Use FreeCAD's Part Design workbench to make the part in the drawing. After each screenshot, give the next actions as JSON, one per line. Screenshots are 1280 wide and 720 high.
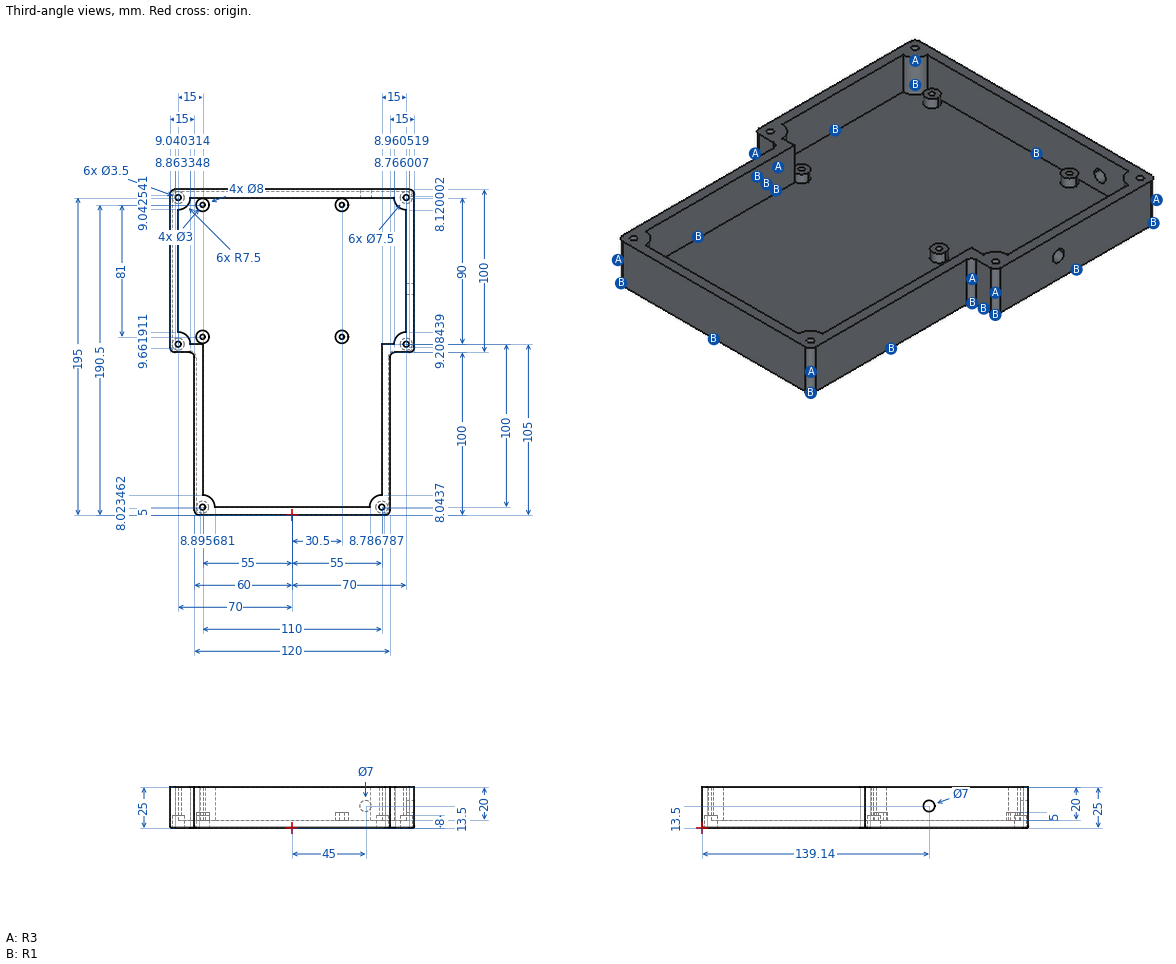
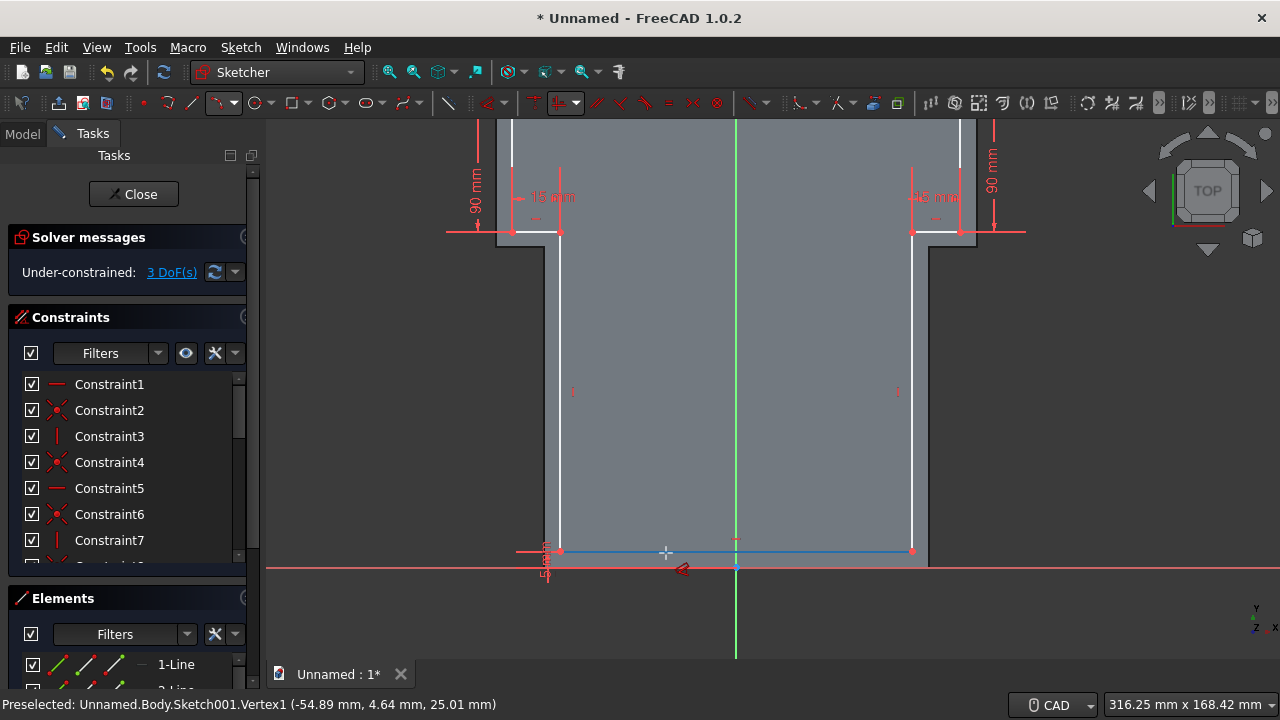
{"action": "left_click", "coordinate": [666, 552]}
{"action": "left_click", "coordinate": [655, 586]}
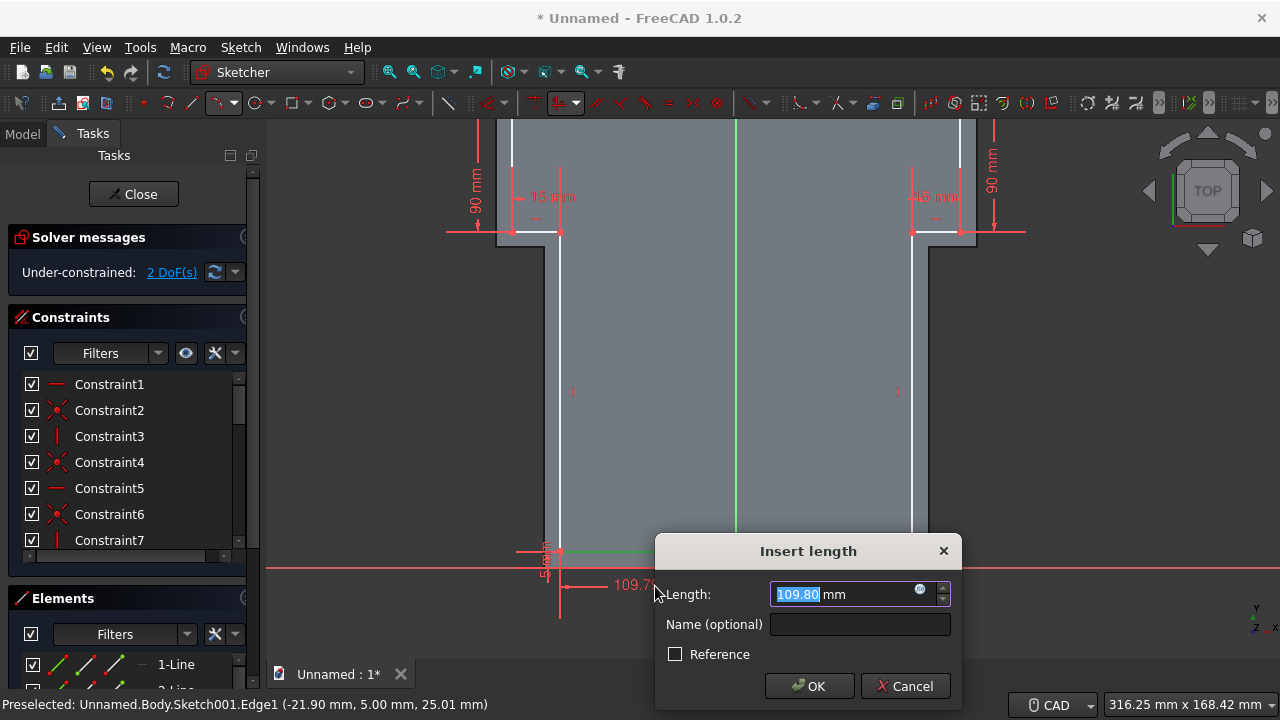
{"action": "type", "text": "110"}
{"action": "key", "text": "Return"}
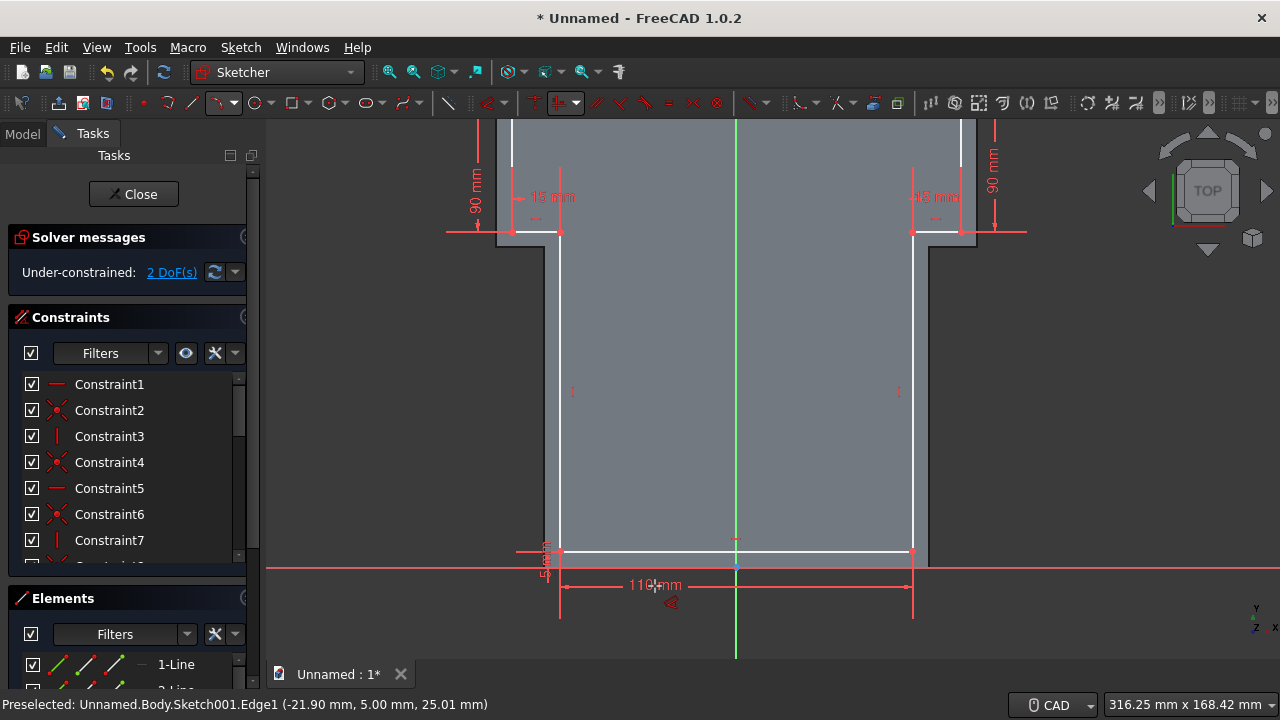
{"action": "left_click", "coordinate": [913, 456]}
{"action": "left_click", "coordinate": [947, 392]}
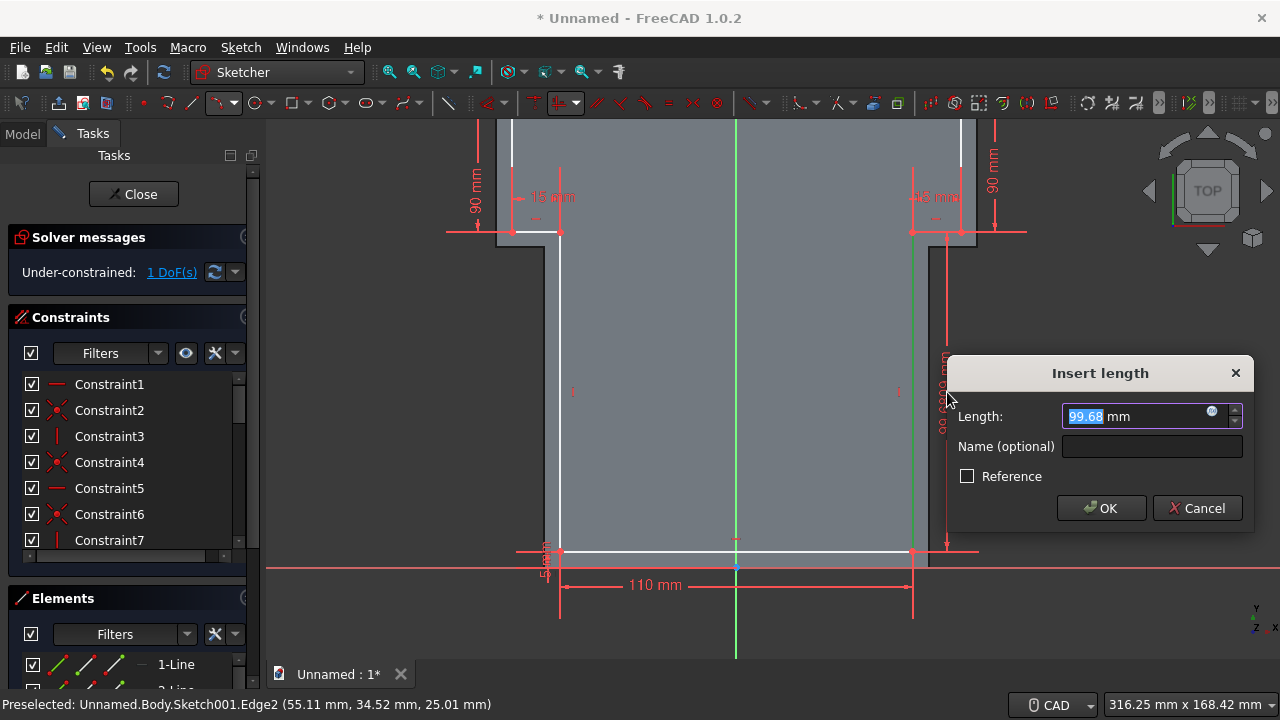
{"action": "type", "text": "100"}
{"action": "key", "text": "Return"}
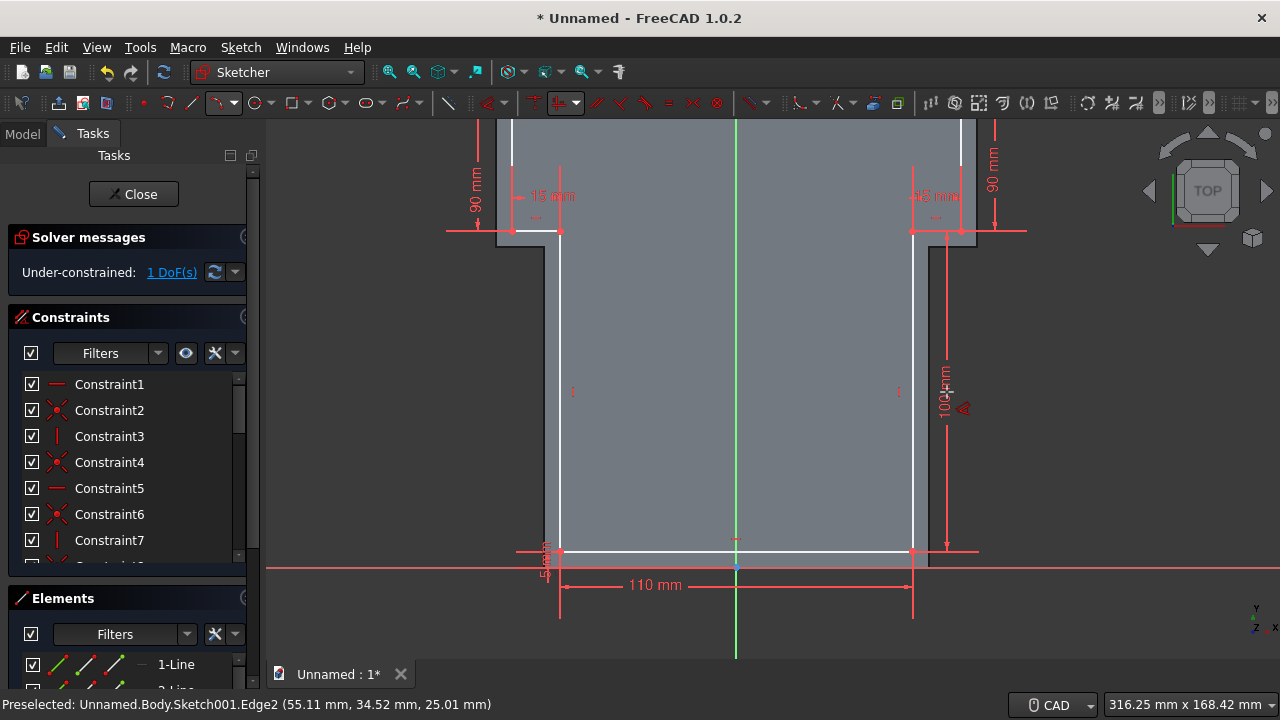
{"action": "left_click", "coordinate": [560, 552]}
{"action": "left_click", "coordinate": [648, 518]}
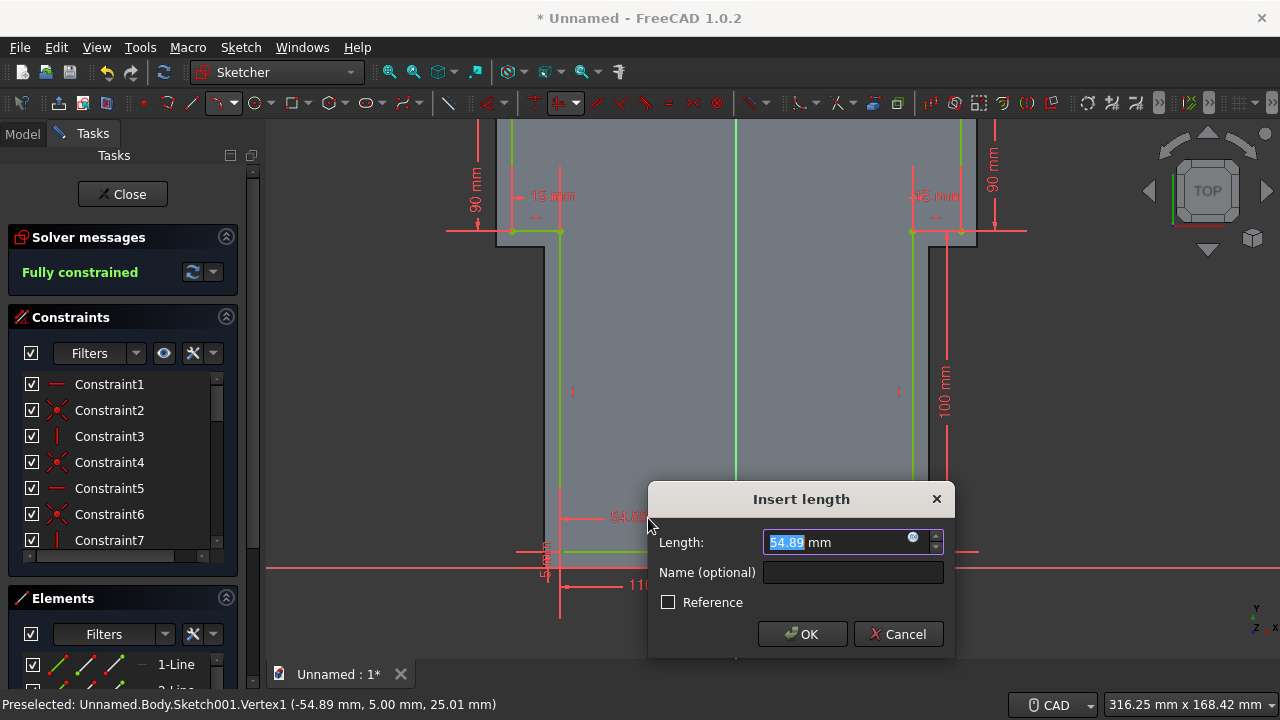
{"action": "type", "text": "55"}
{"action": "key", "text": "Return"}
{"action": "key", "text": "Escape"}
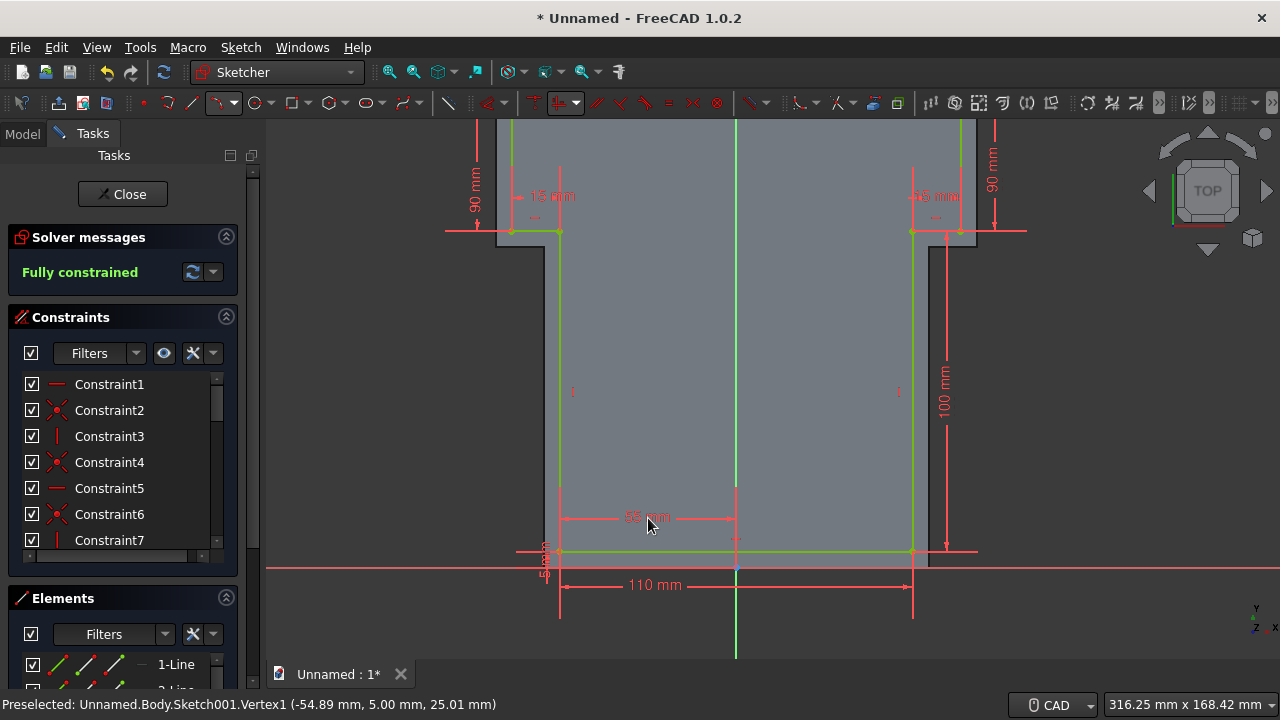
{"action": "left_click", "coordinate": [123, 194]}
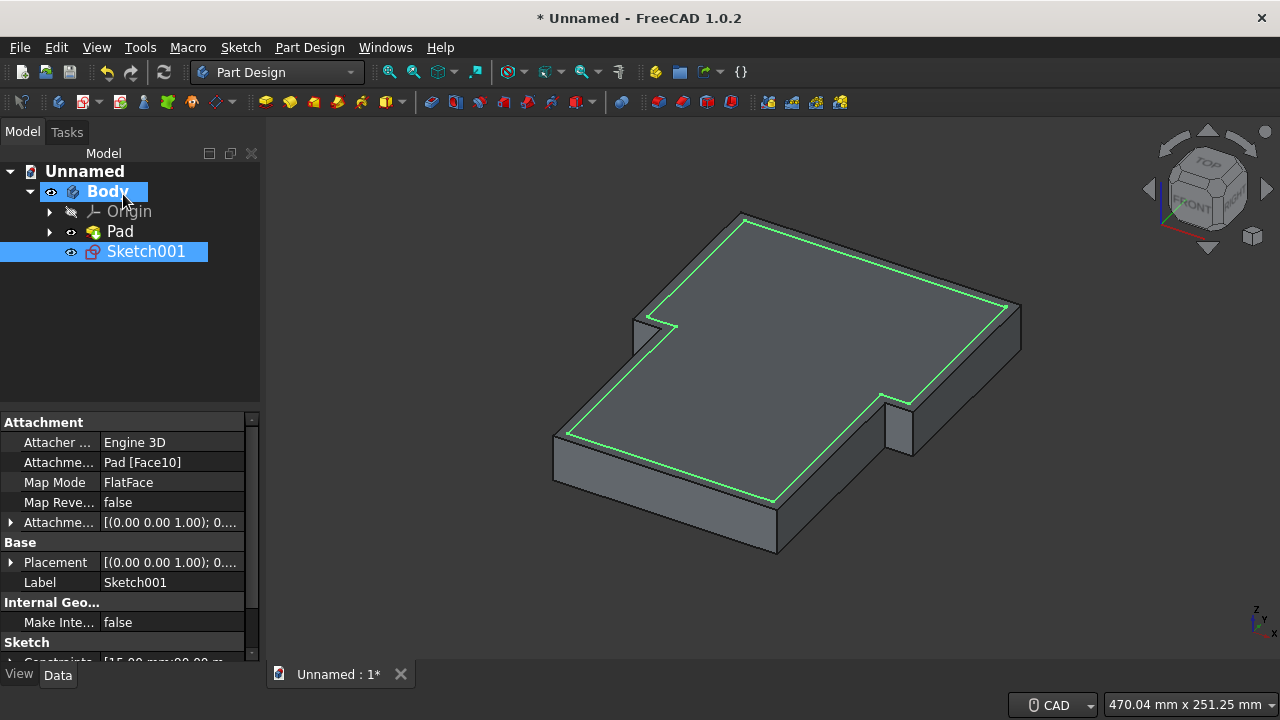
{"action": "left_click", "coordinate": [432, 102]}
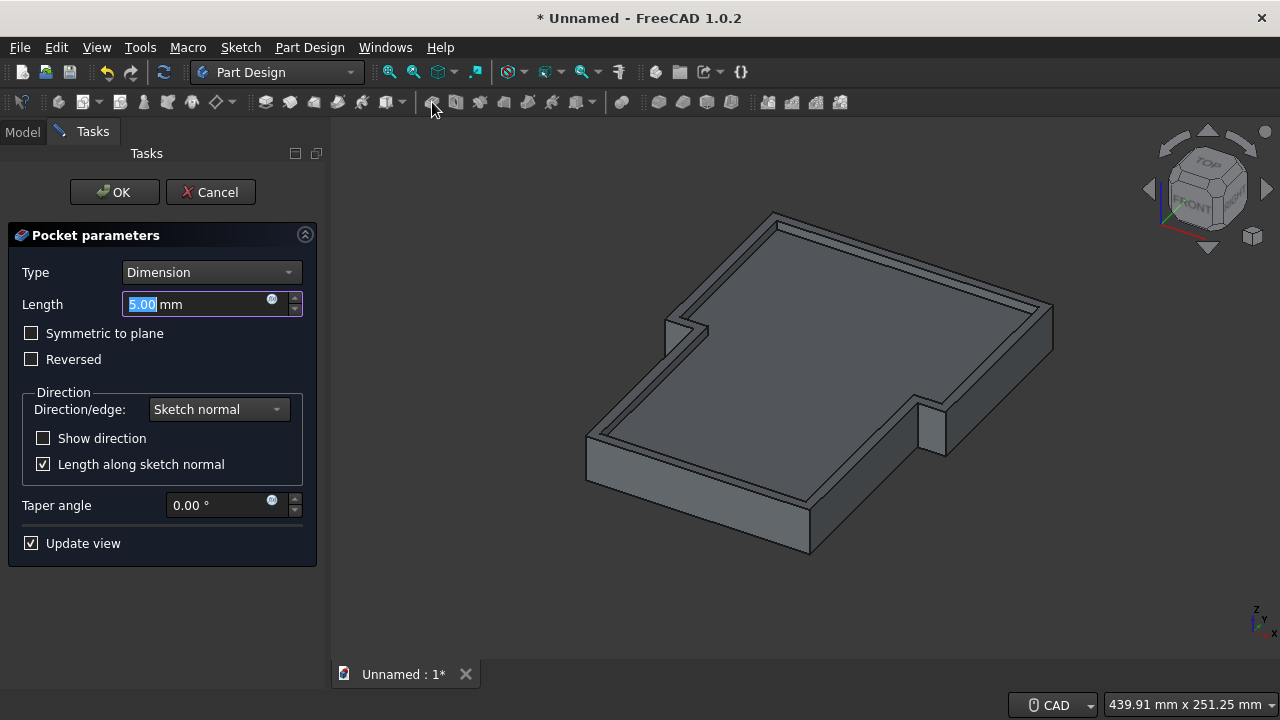
{"action": "type", "text": "20"}
{"action": "key", "text": "Tab"}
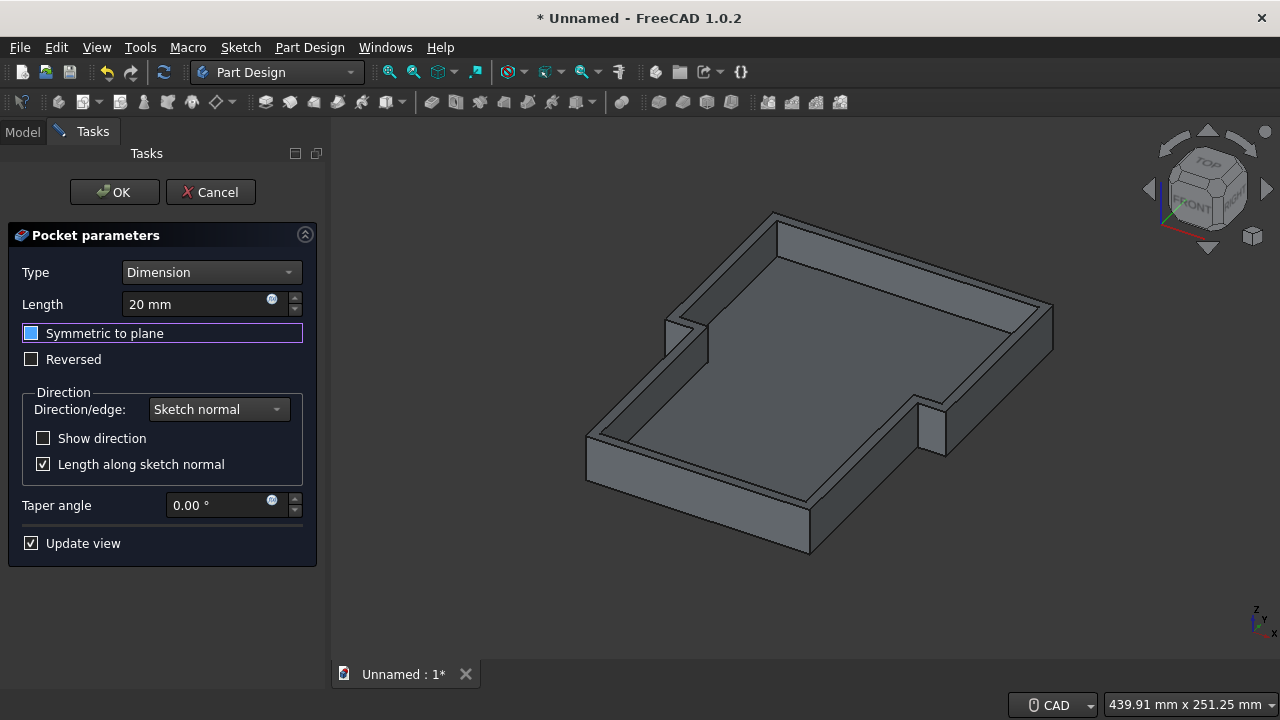
{"action": "left_click", "coordinate": [115, 192]}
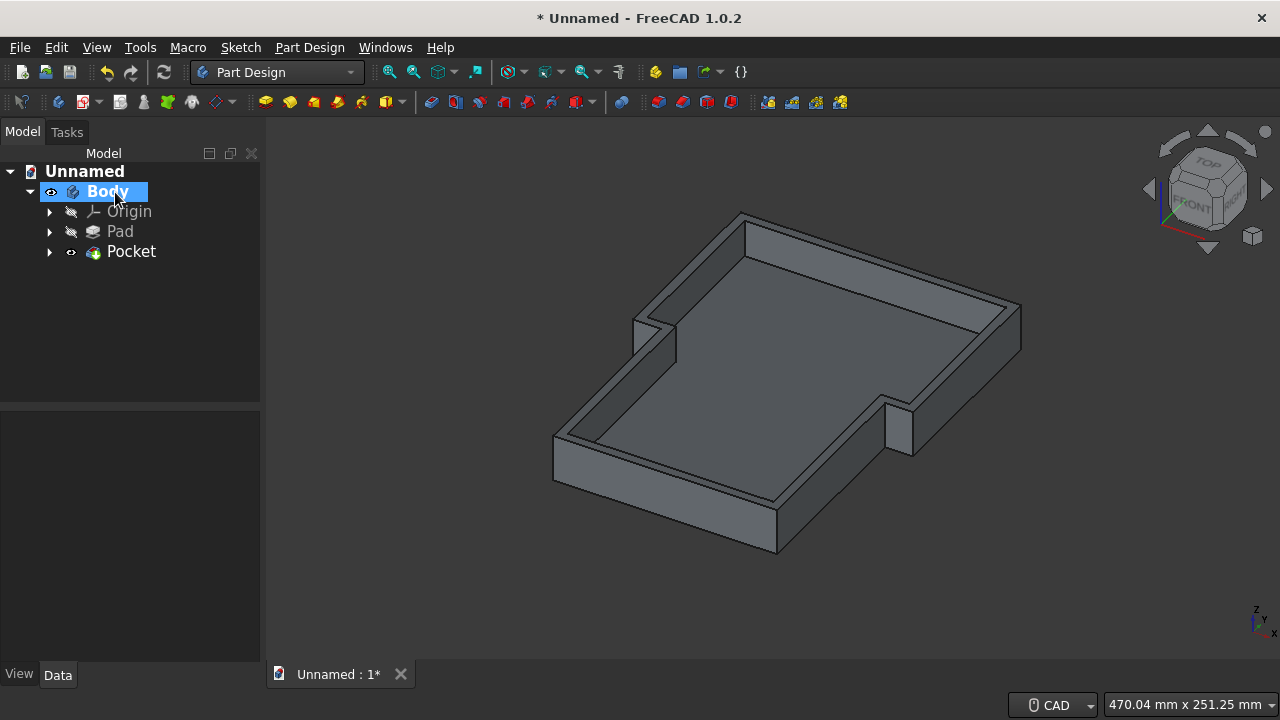
{"action": "left_click", "coordinate": [913, 433]}